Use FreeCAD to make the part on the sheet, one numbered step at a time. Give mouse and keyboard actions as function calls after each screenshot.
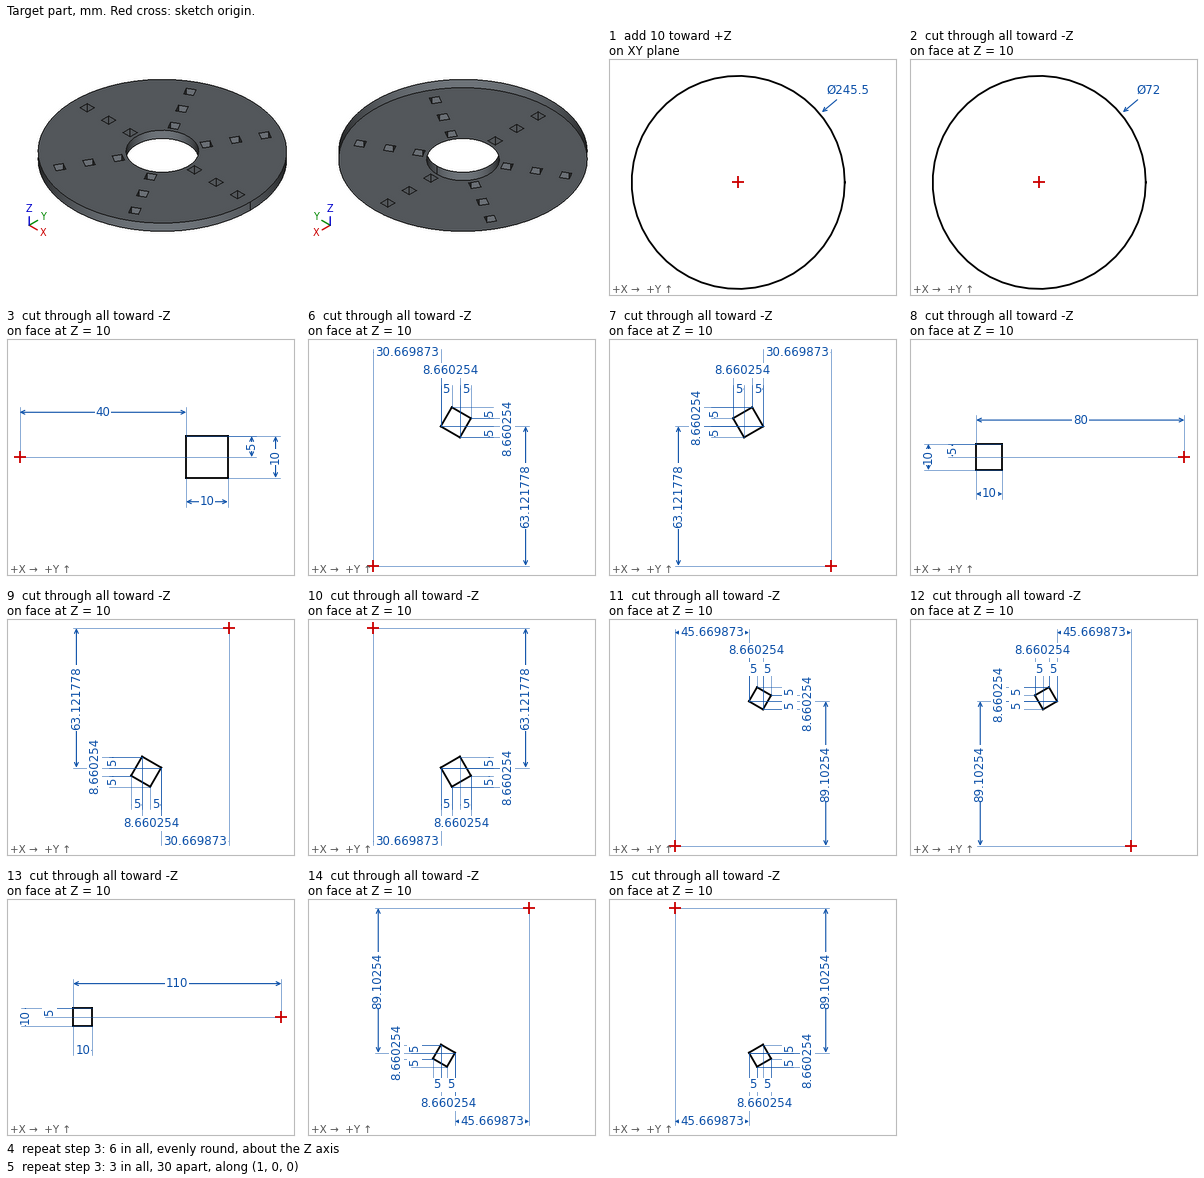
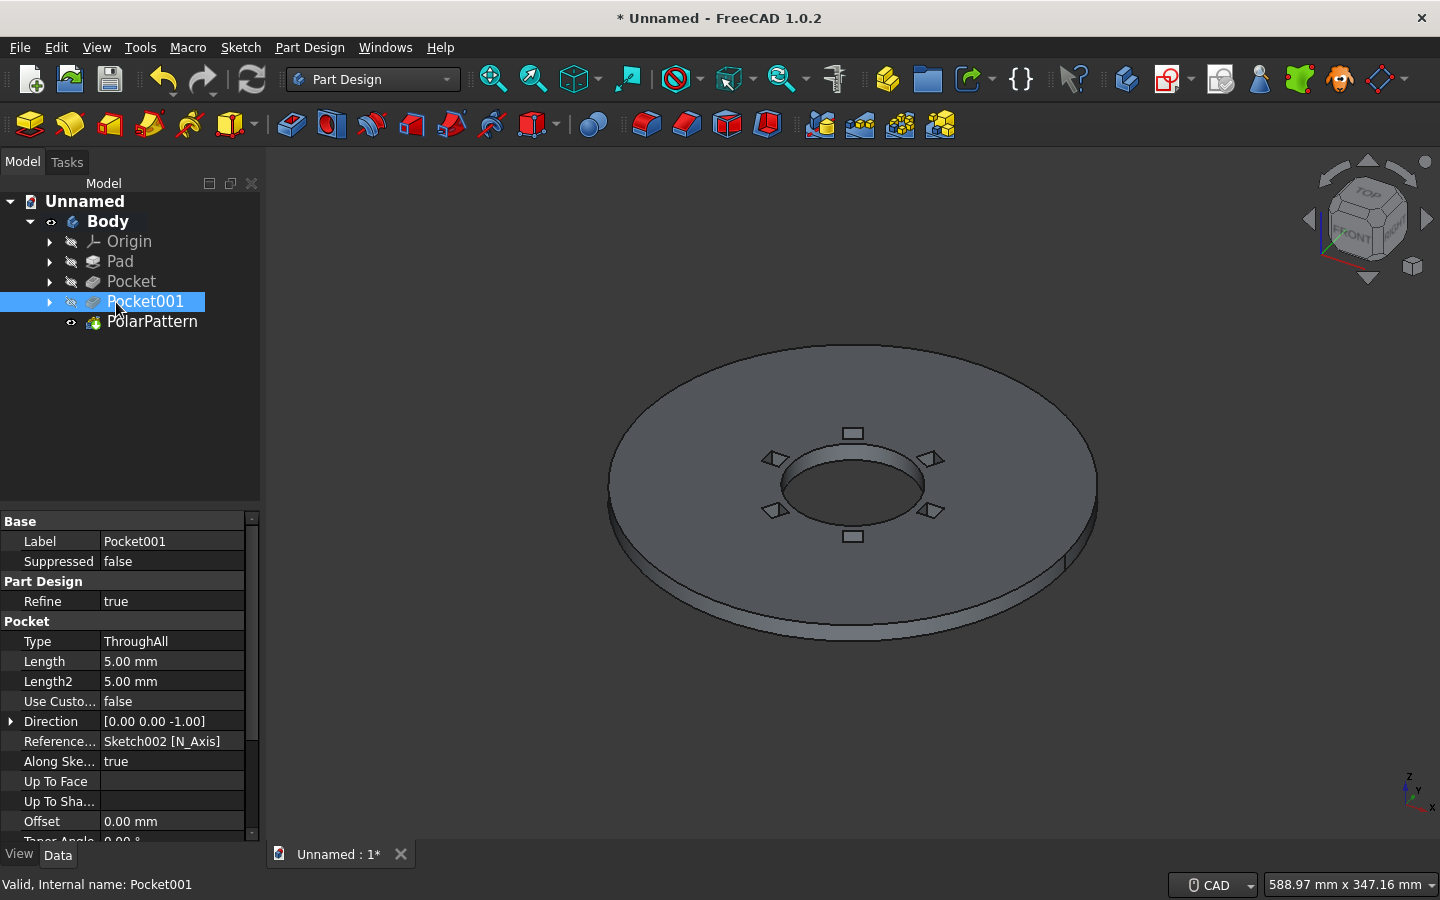
click(860, 124)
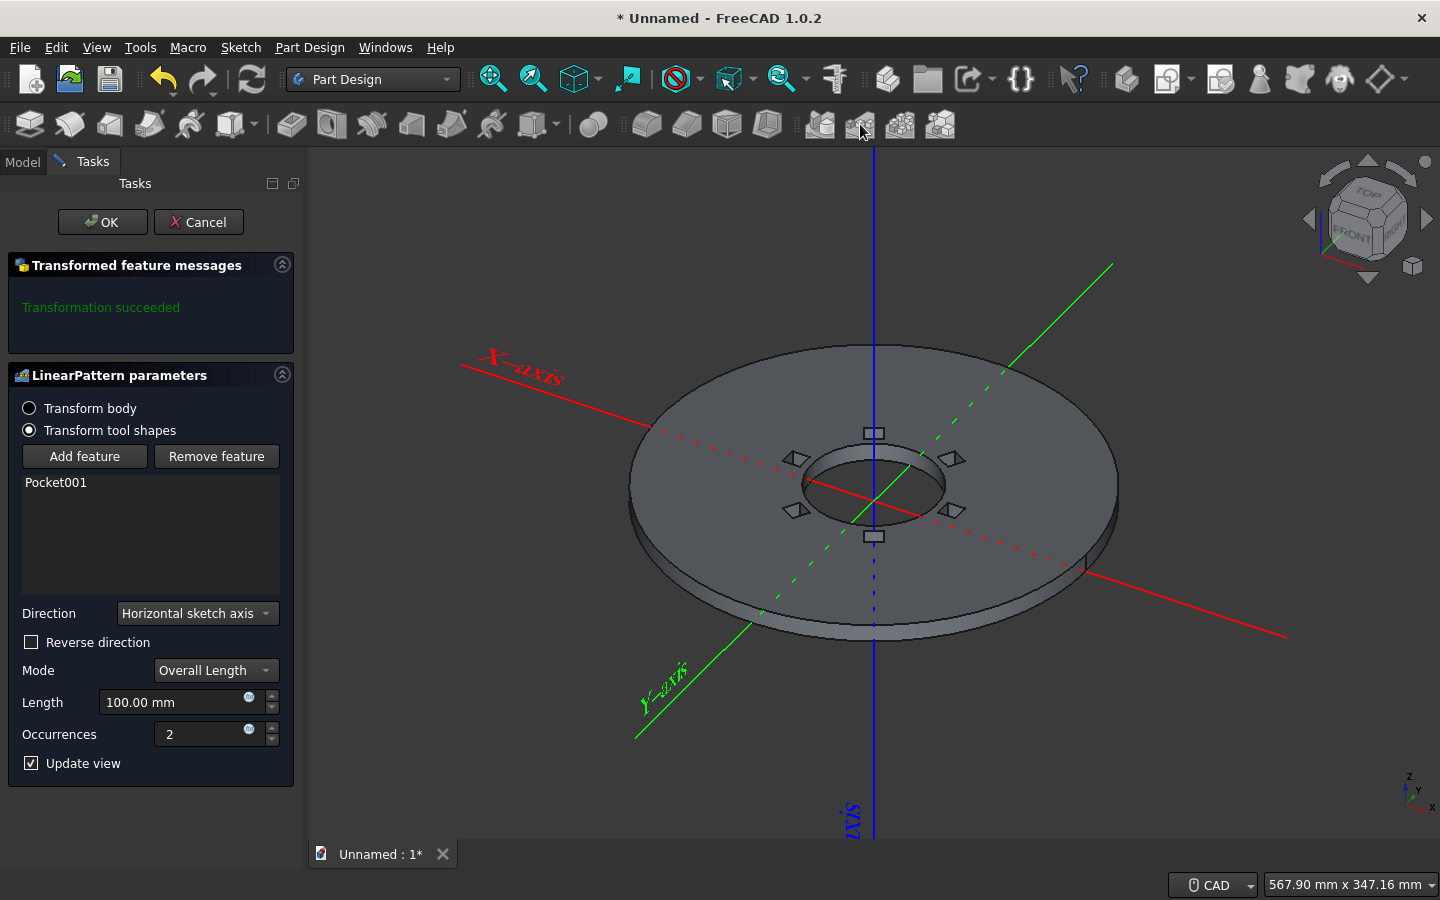
click(198, 614)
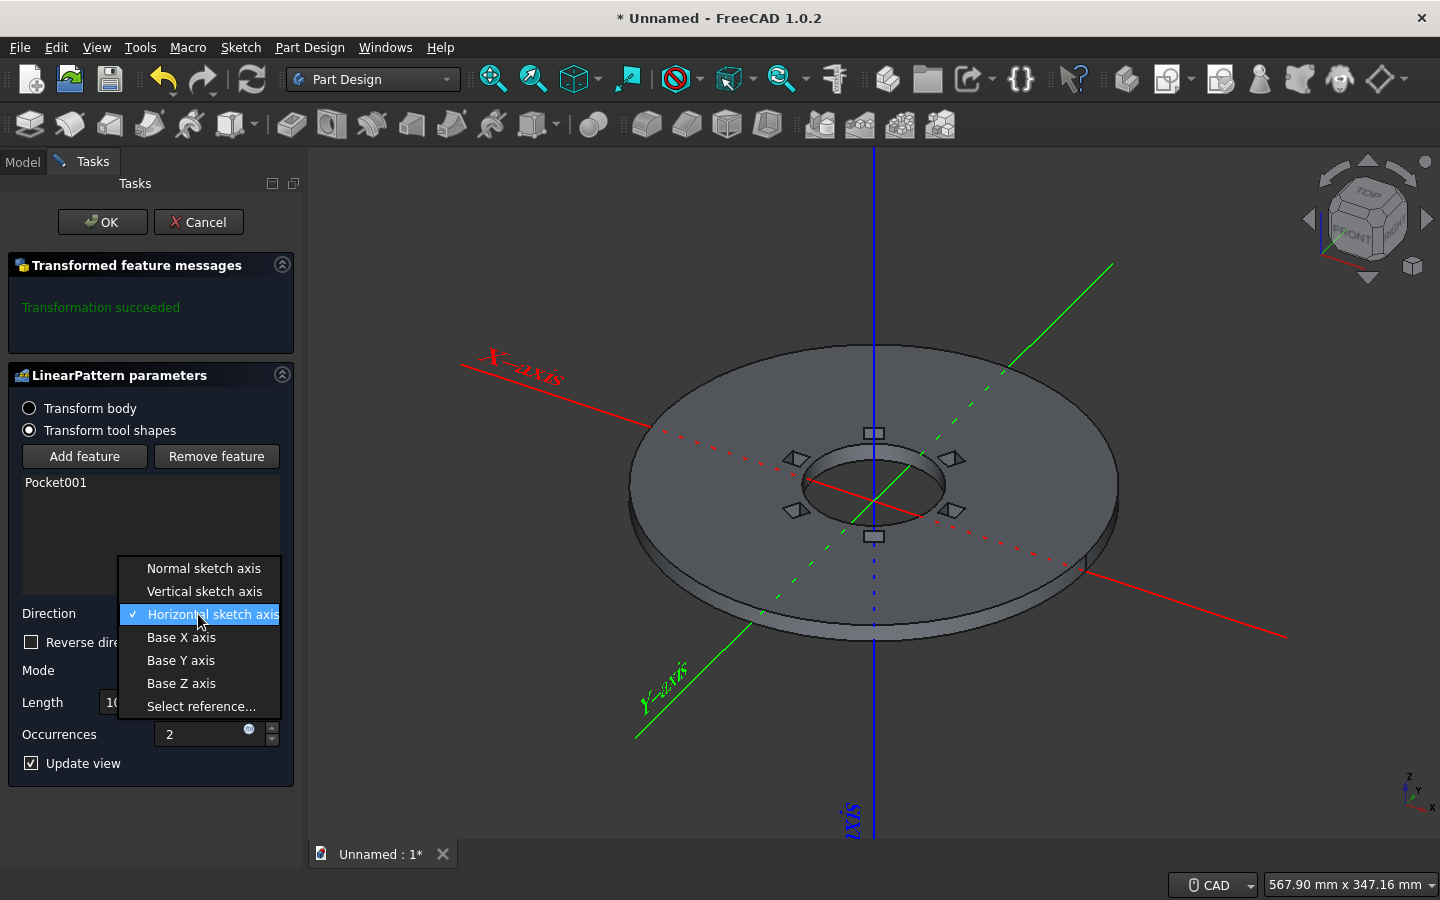
click(198, 638)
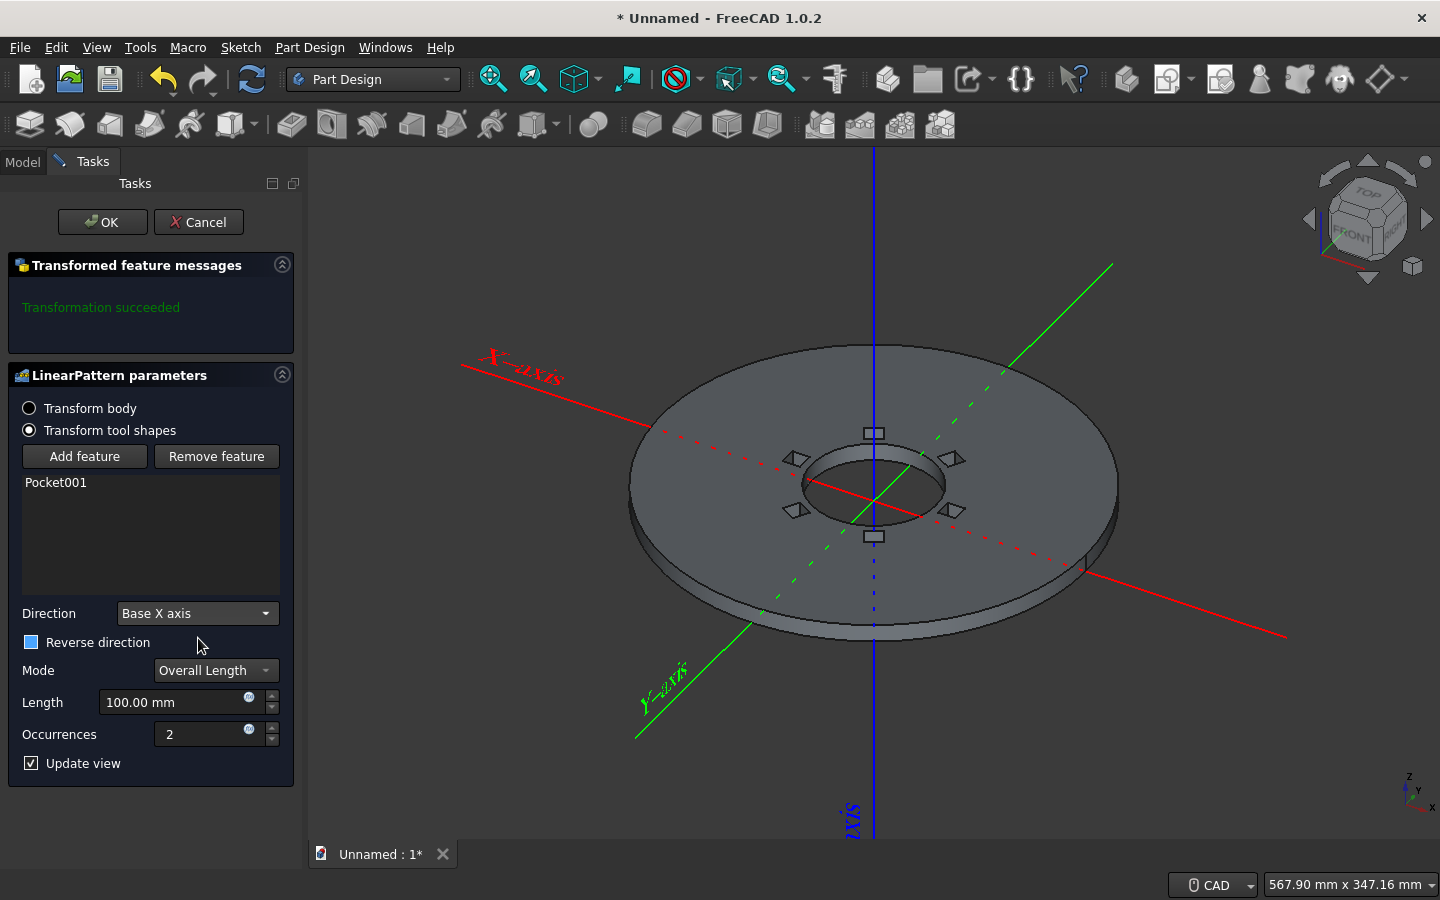
click(217, 670)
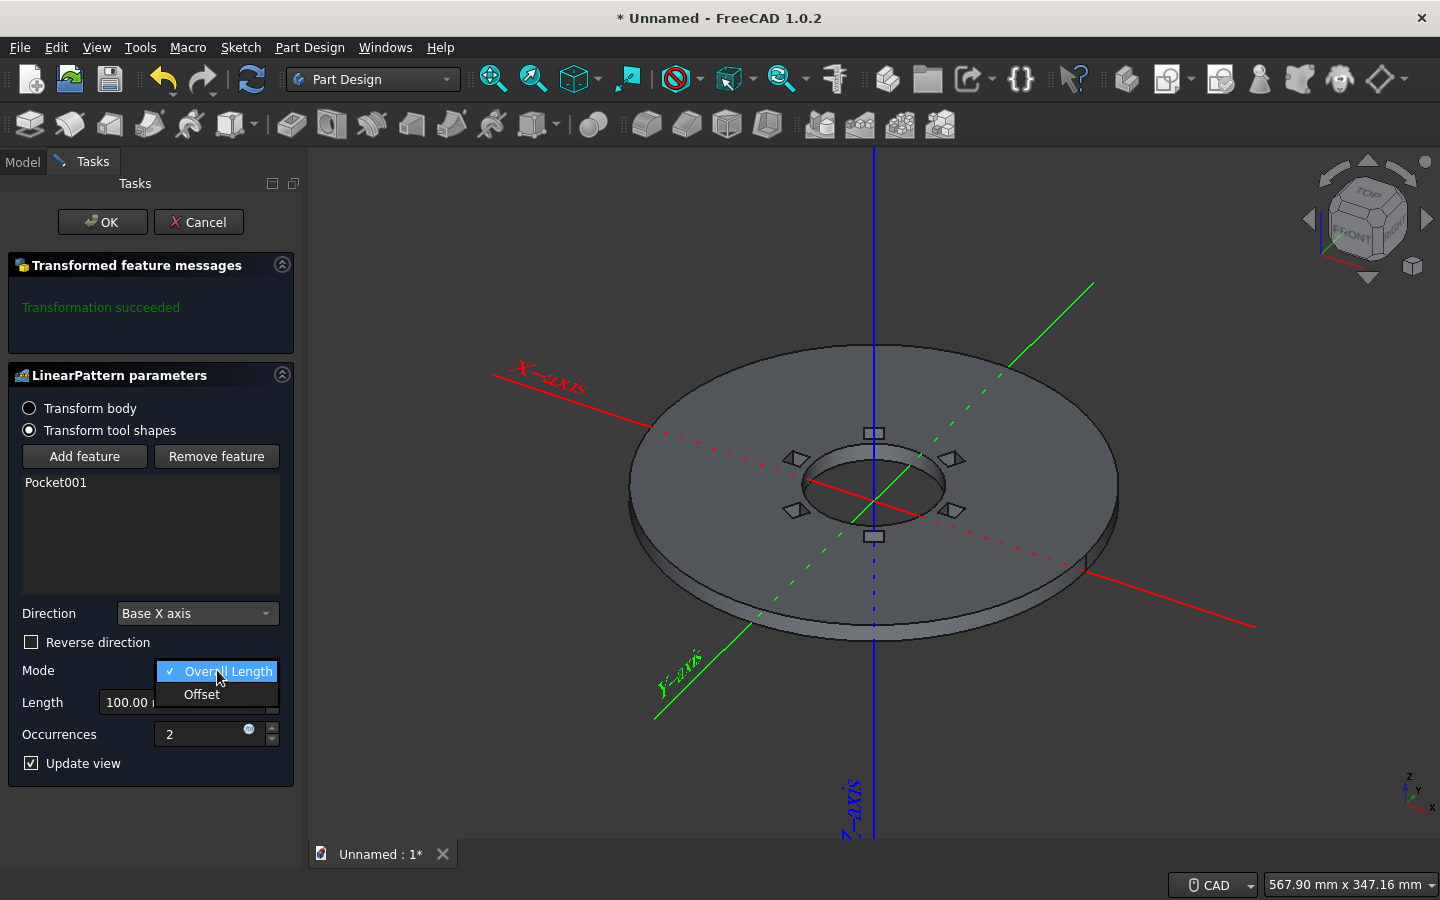
click(216, 694)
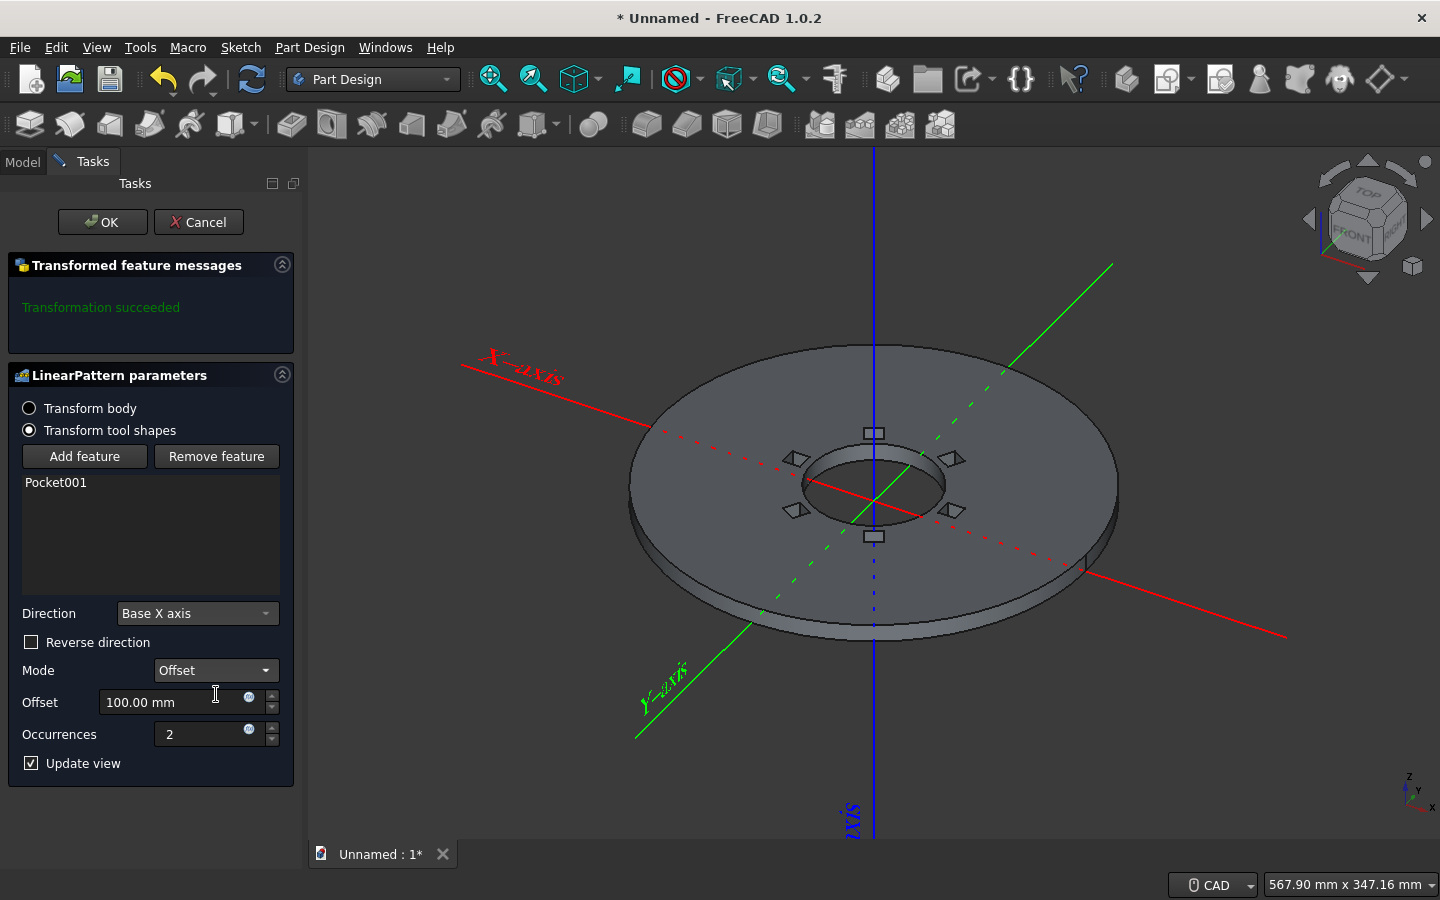
triple_click(182, 702)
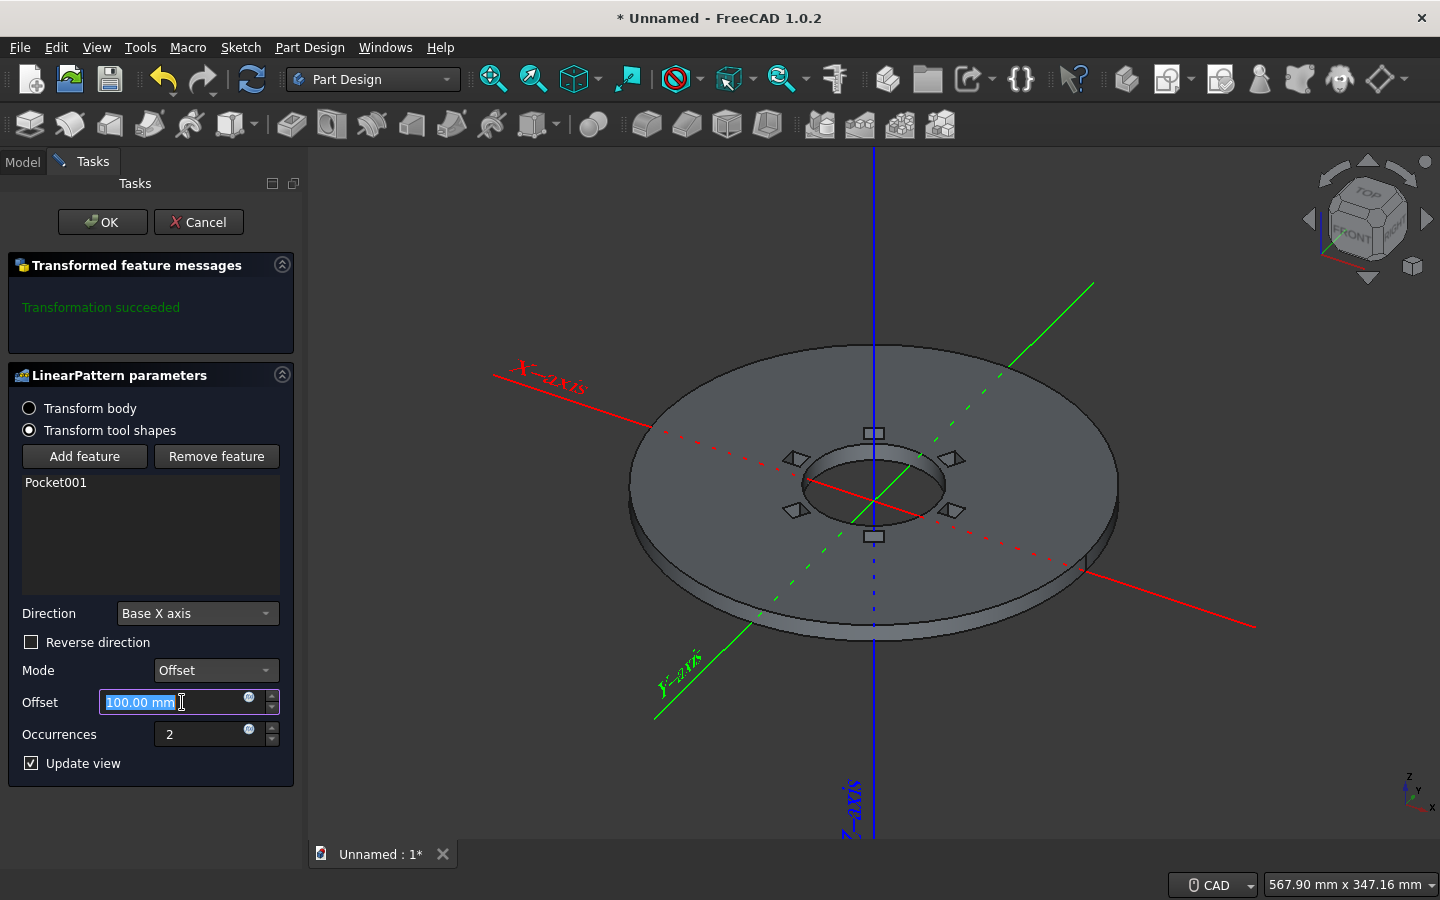
text(30)
key(Tab)